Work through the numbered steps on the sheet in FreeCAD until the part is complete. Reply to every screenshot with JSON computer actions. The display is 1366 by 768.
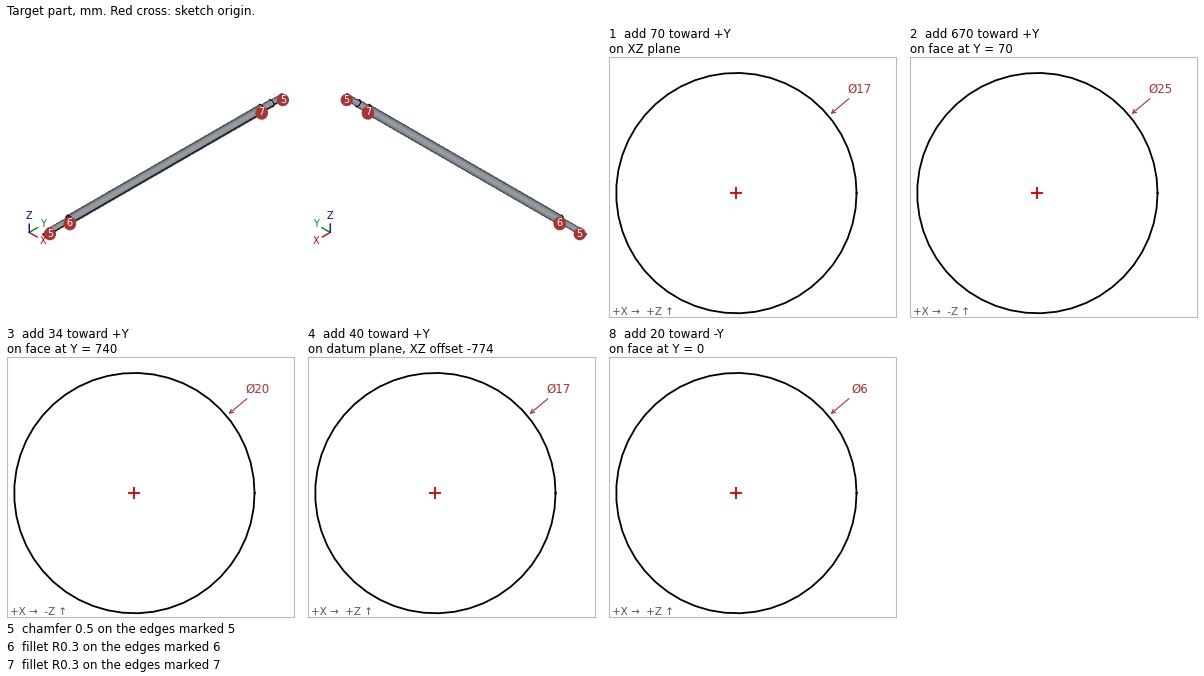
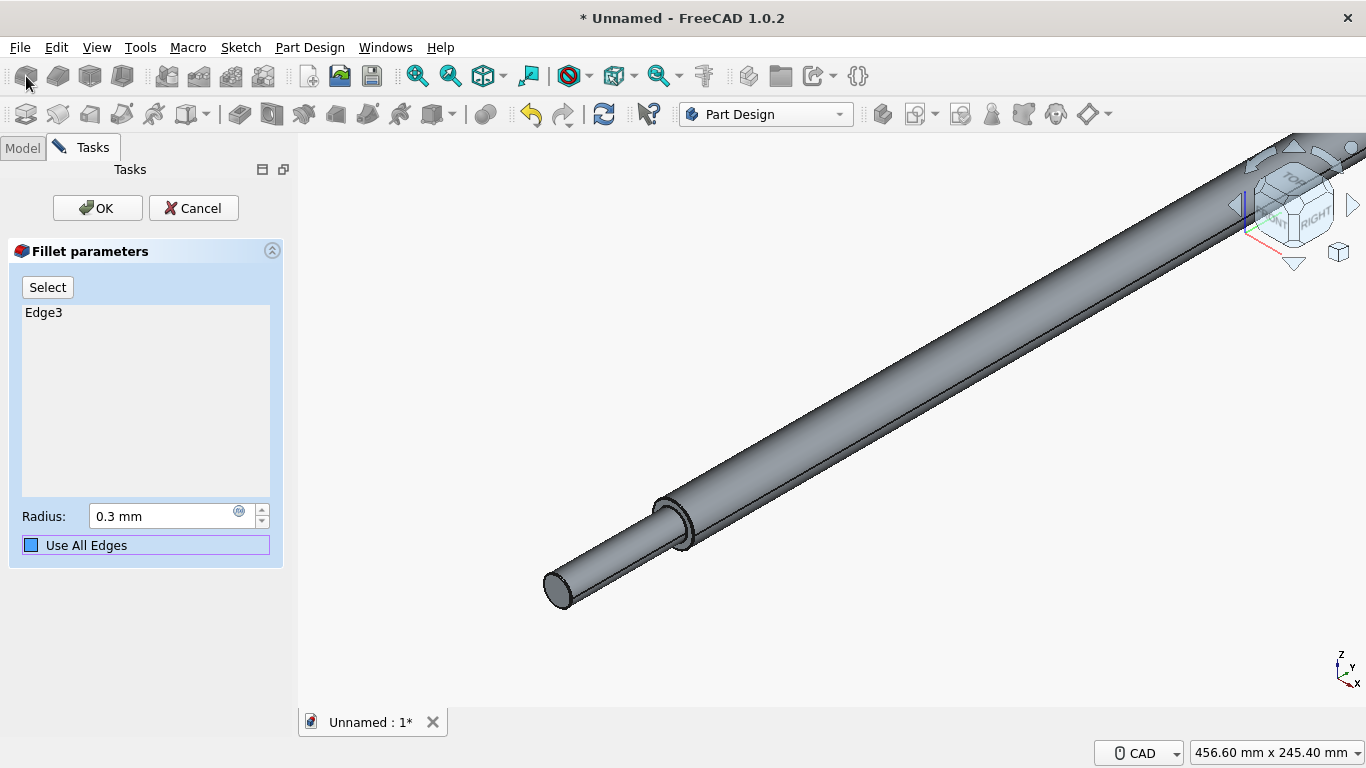
{"action": "left_click", "coordinate": [98, 208]}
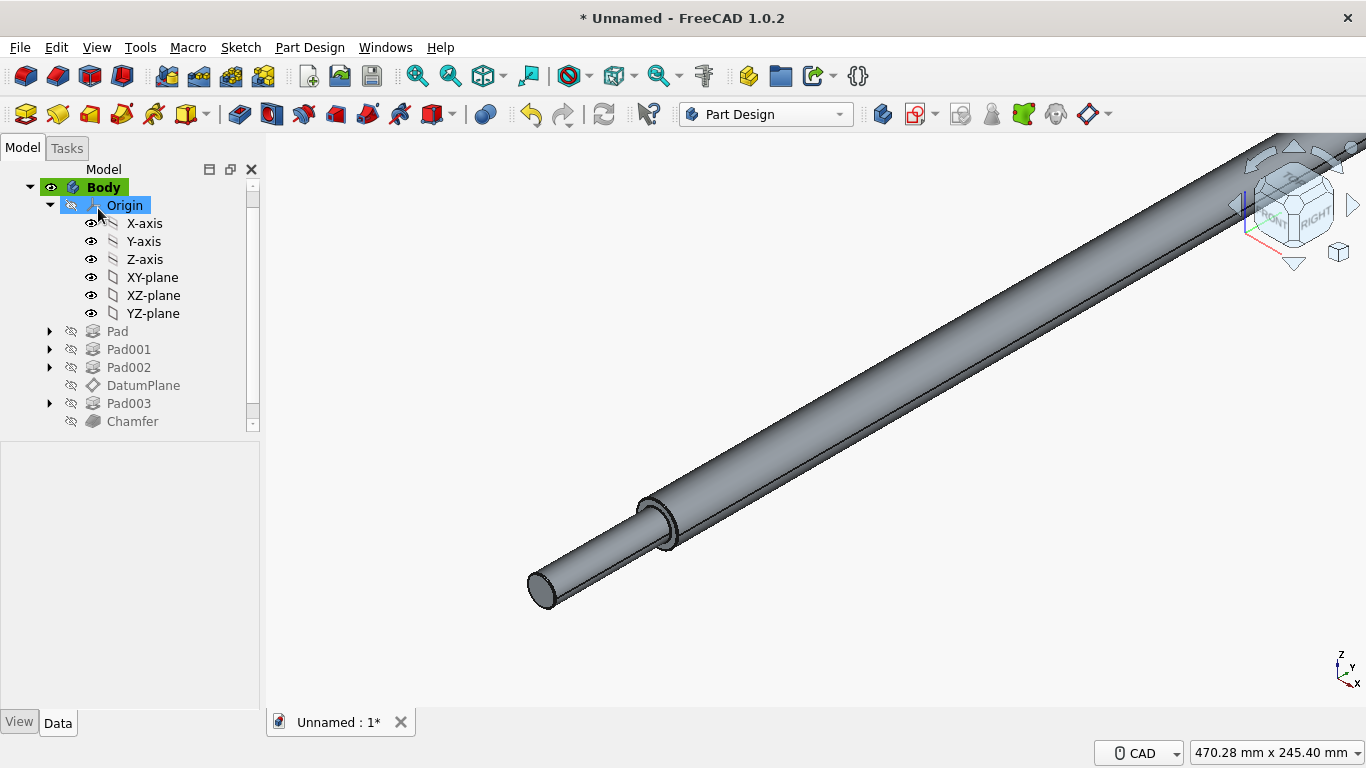
{"action": "left_click", "coordinate": [418, 76]}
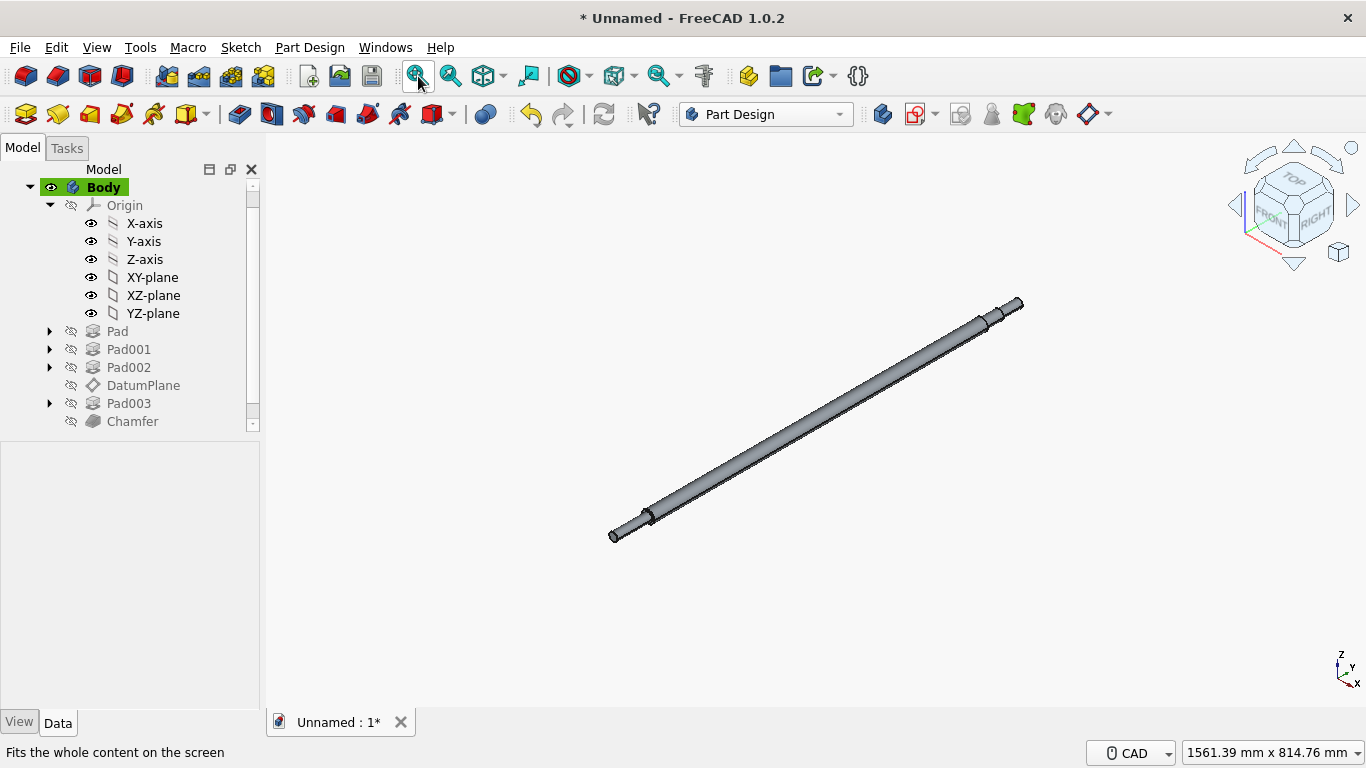
{"action": "key", "text": "2"}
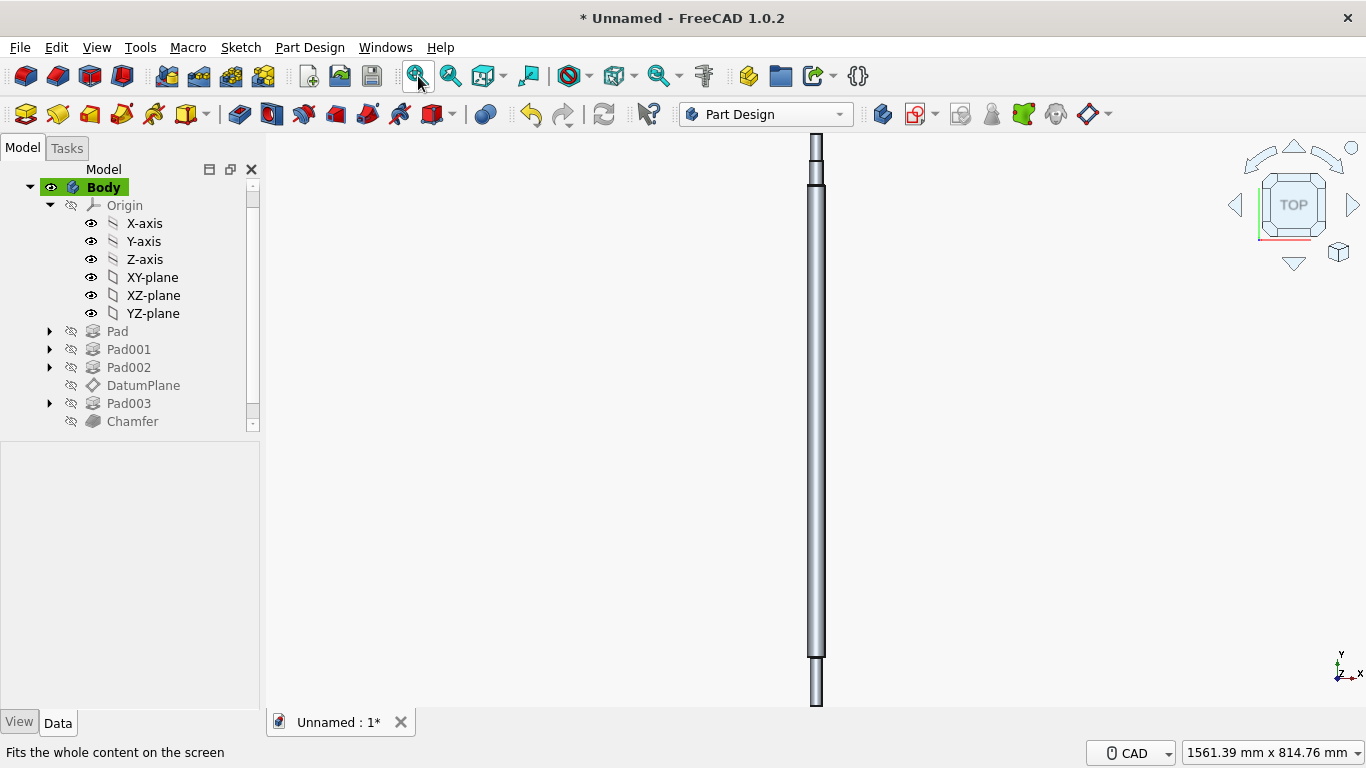
{"action": "left_click", "coordinate": [418, 76]}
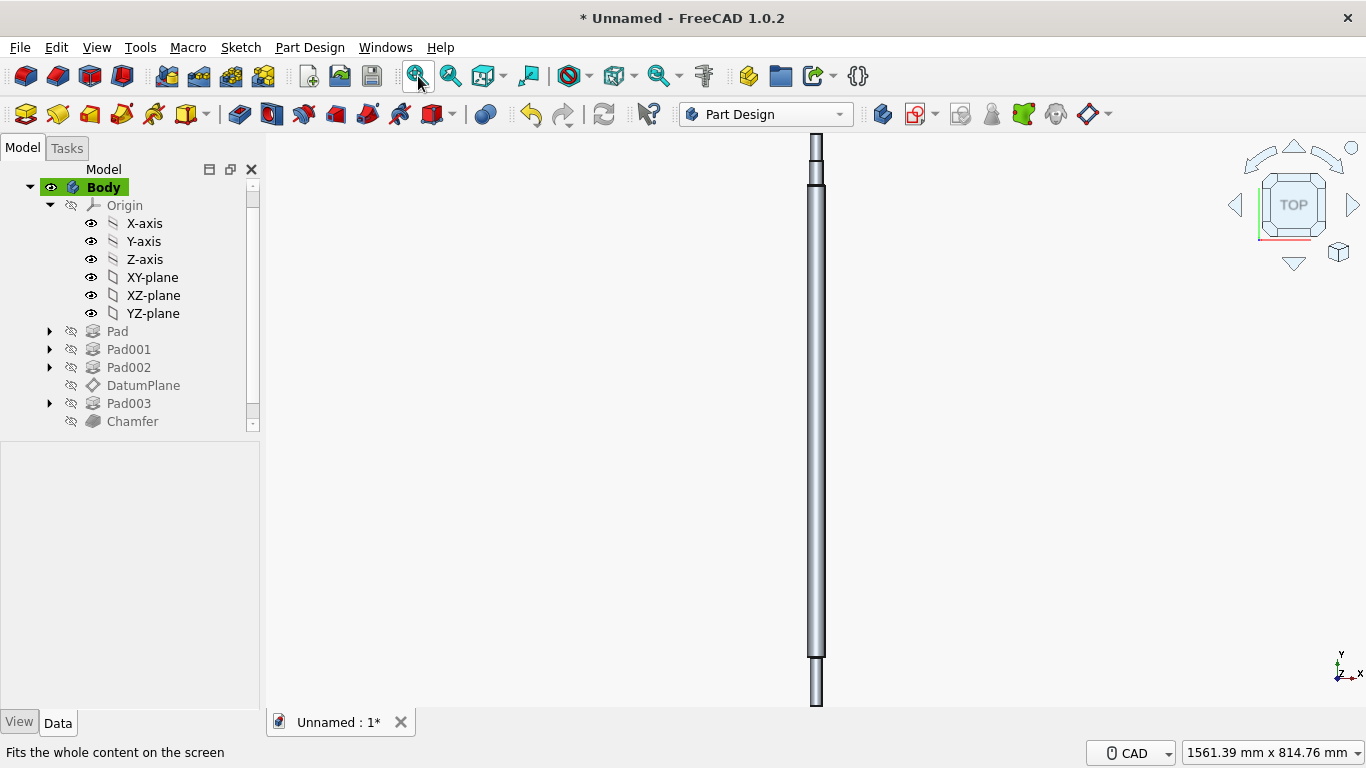
{"action": "key", "text": "0"}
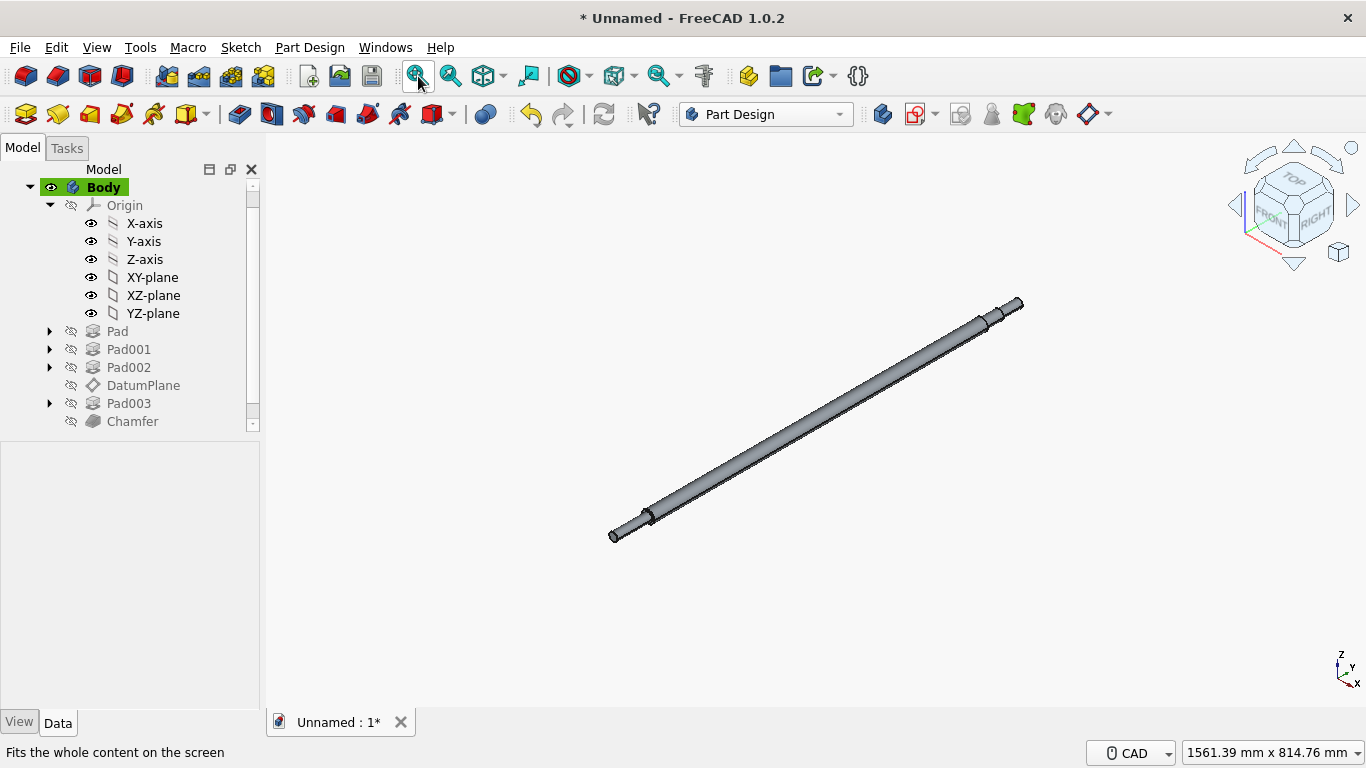
{"action": "left_click", "coordinate": [418, 76]}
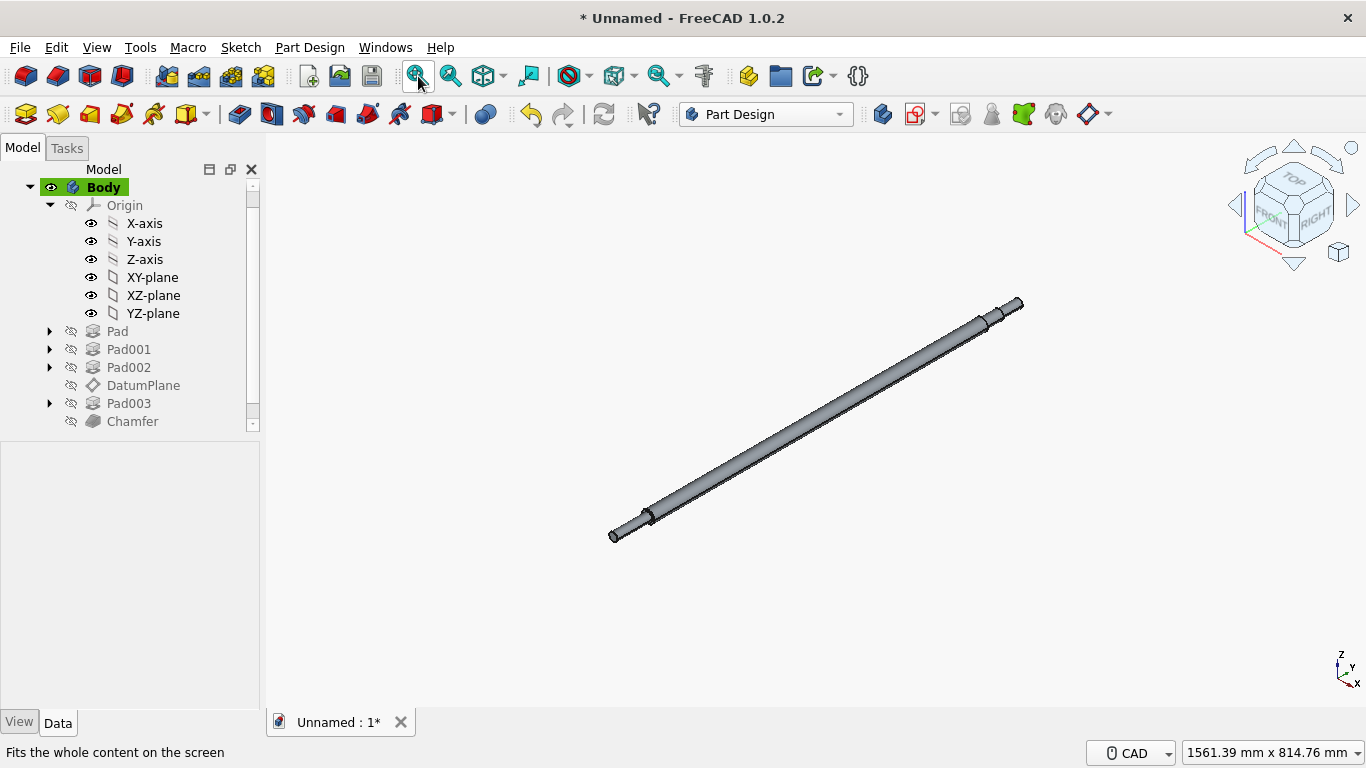
{"action": "key", "text": "1"}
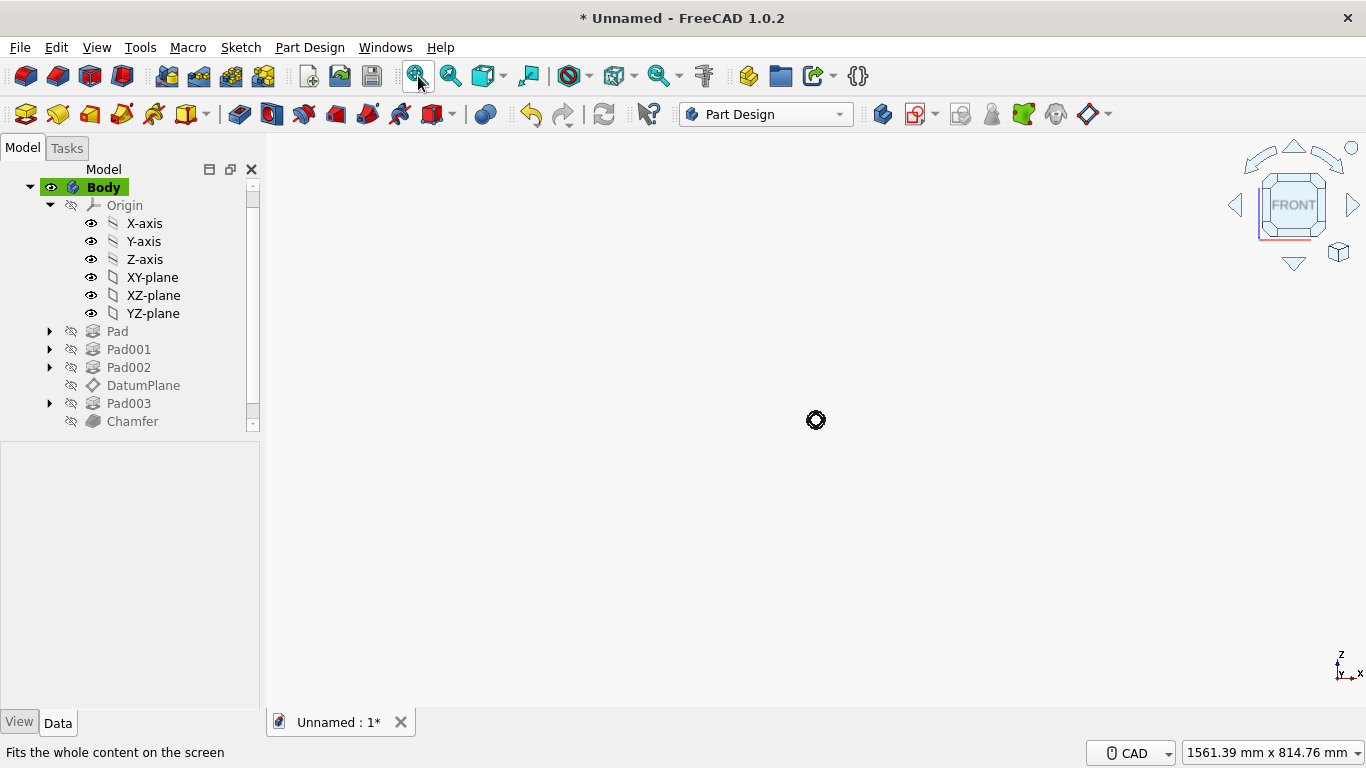
{"action": "left_click", "coordinate": [418, 76]}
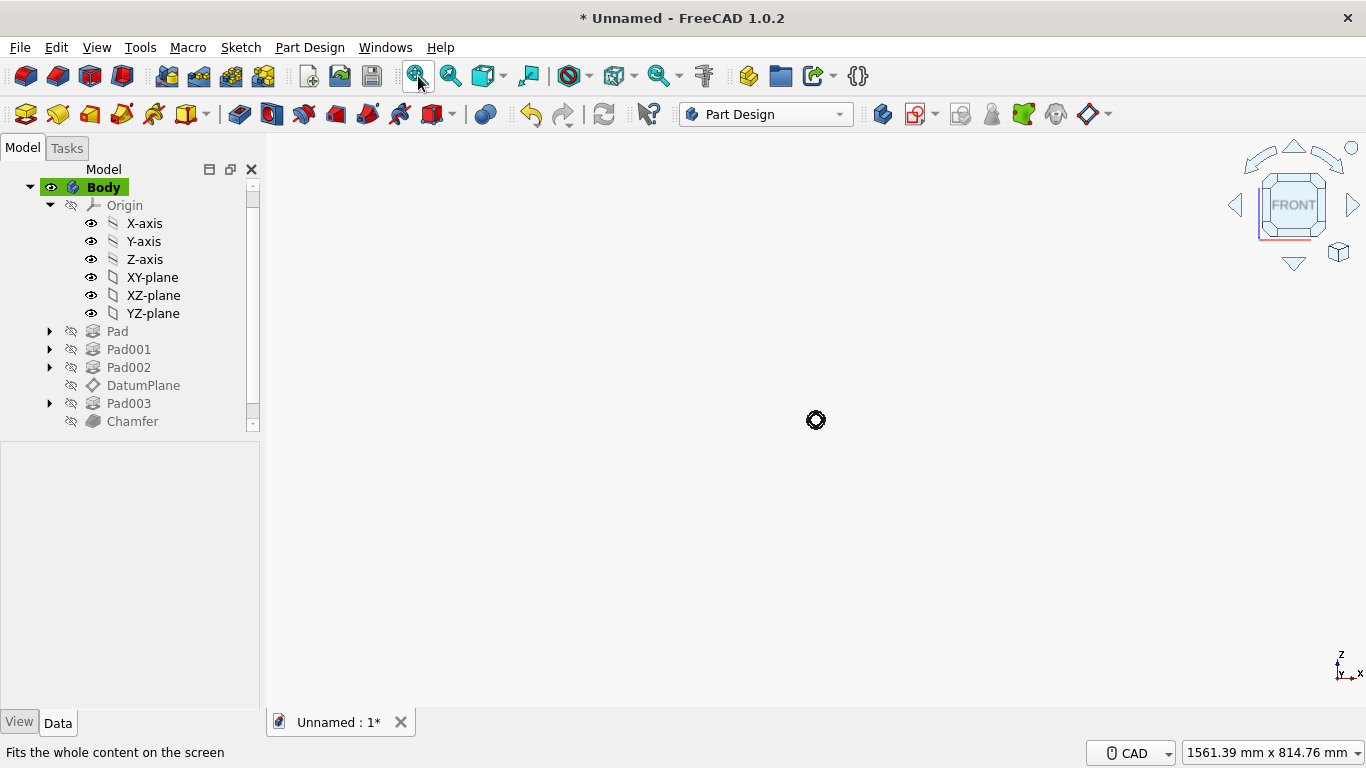
{"action": "key", "text": "3"}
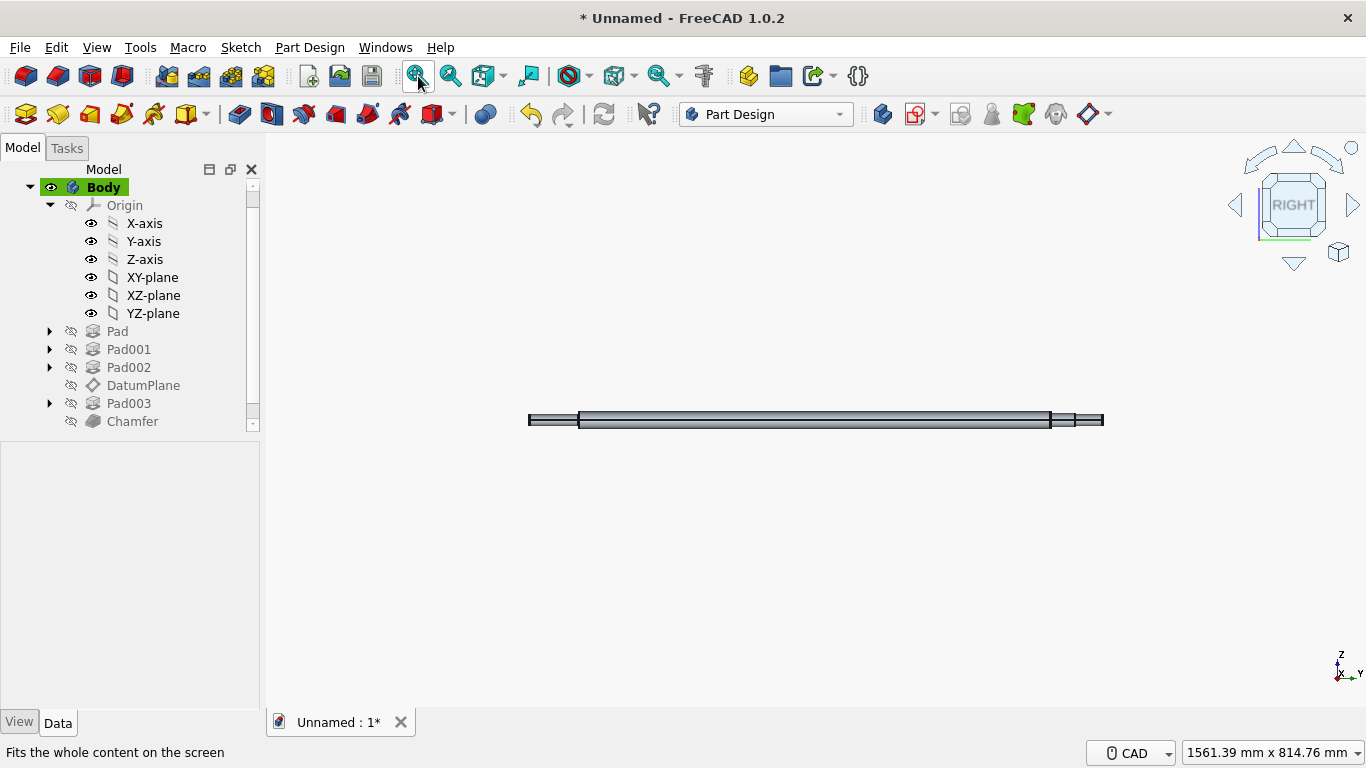
{"action": "key", "text": "5"}